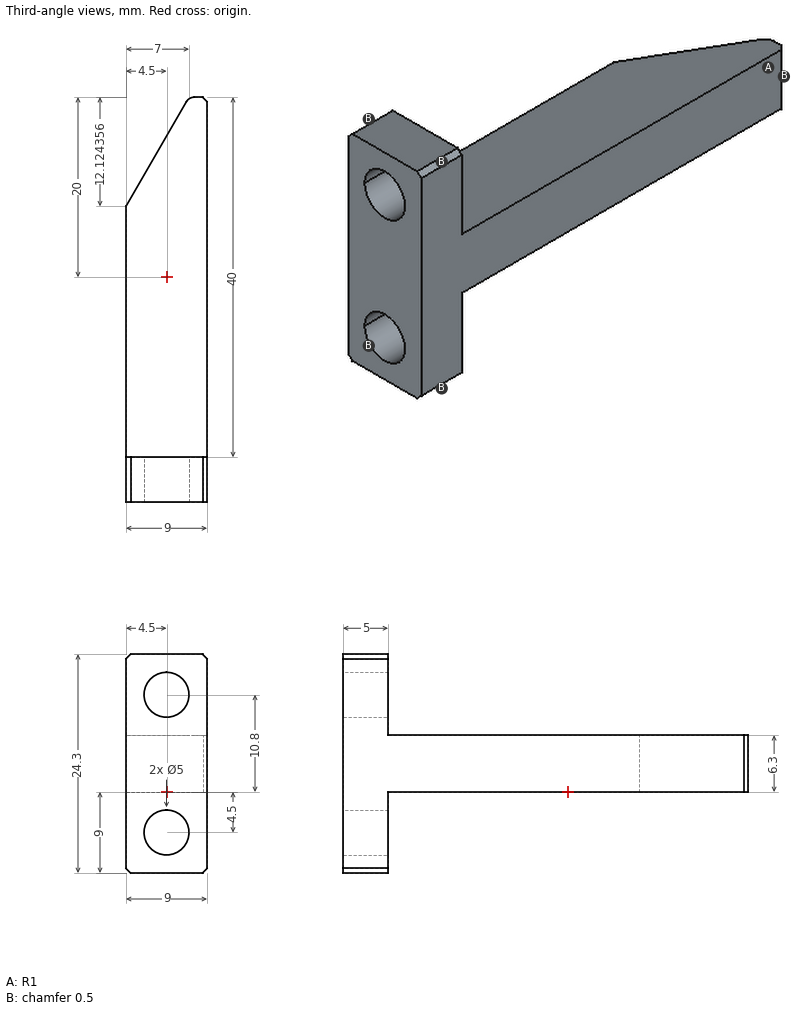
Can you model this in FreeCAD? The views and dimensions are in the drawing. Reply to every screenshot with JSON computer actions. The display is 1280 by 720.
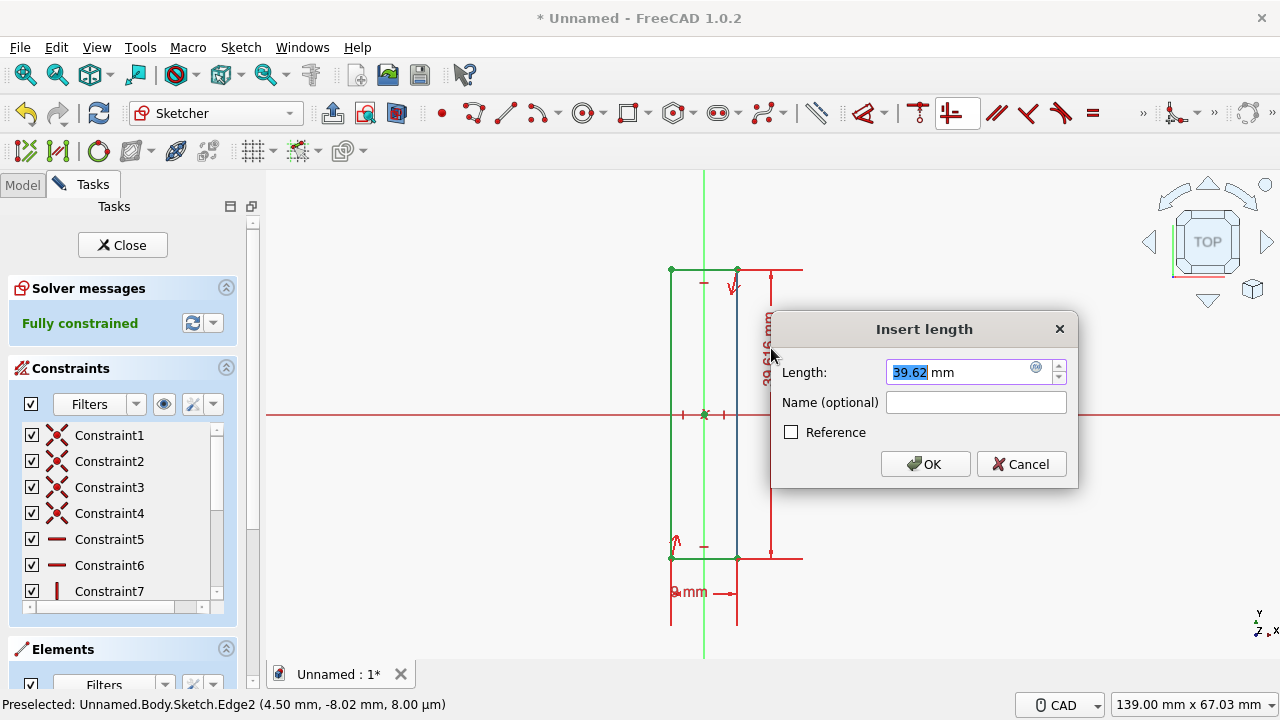
{"action": "type", "text": "40"}
{"action": "key", "text": "Return"}
{"action": "key", "text": "Escape"}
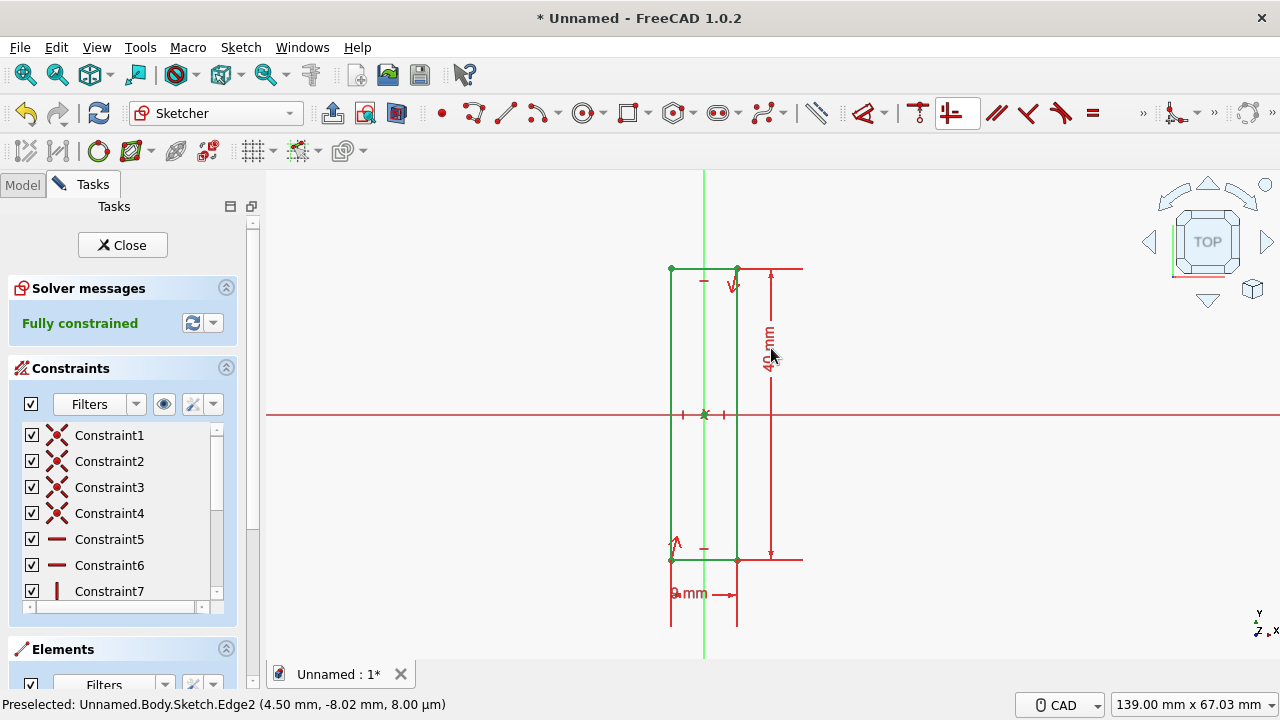
{"action": "left_click", "coordinate": [123, 245]}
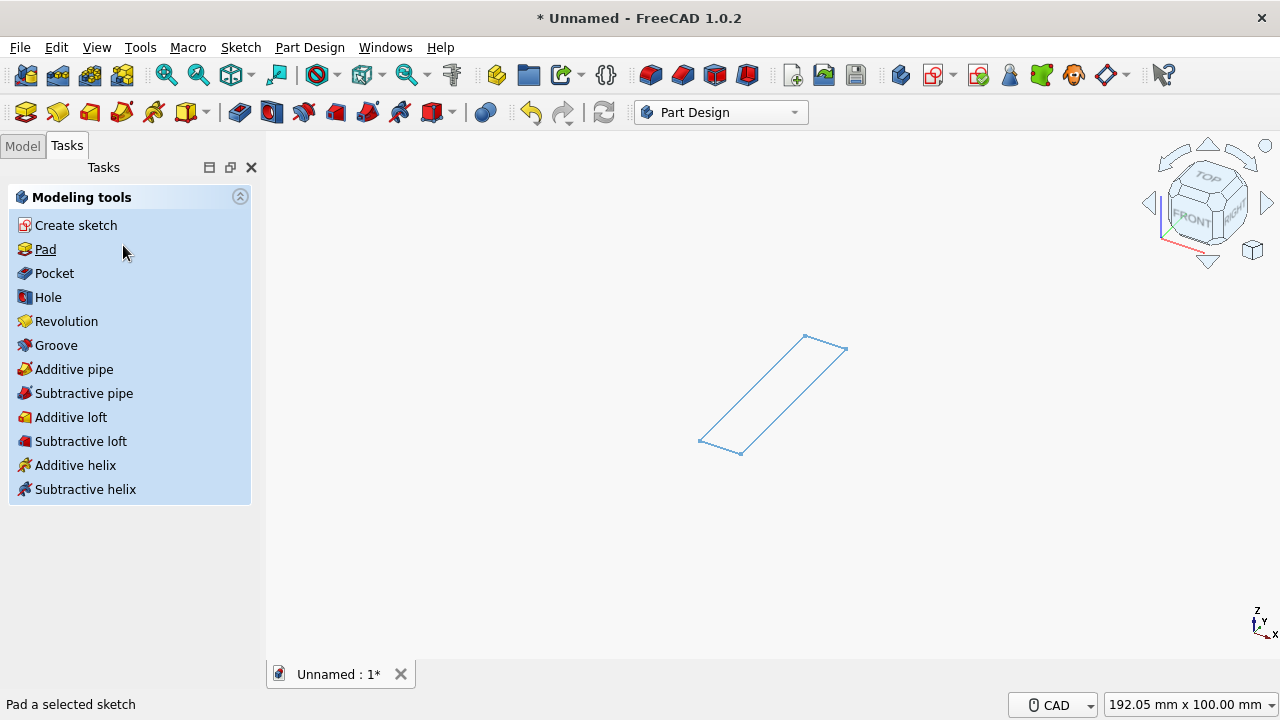
{"action": "left_click", "coordinate": [26, 112]}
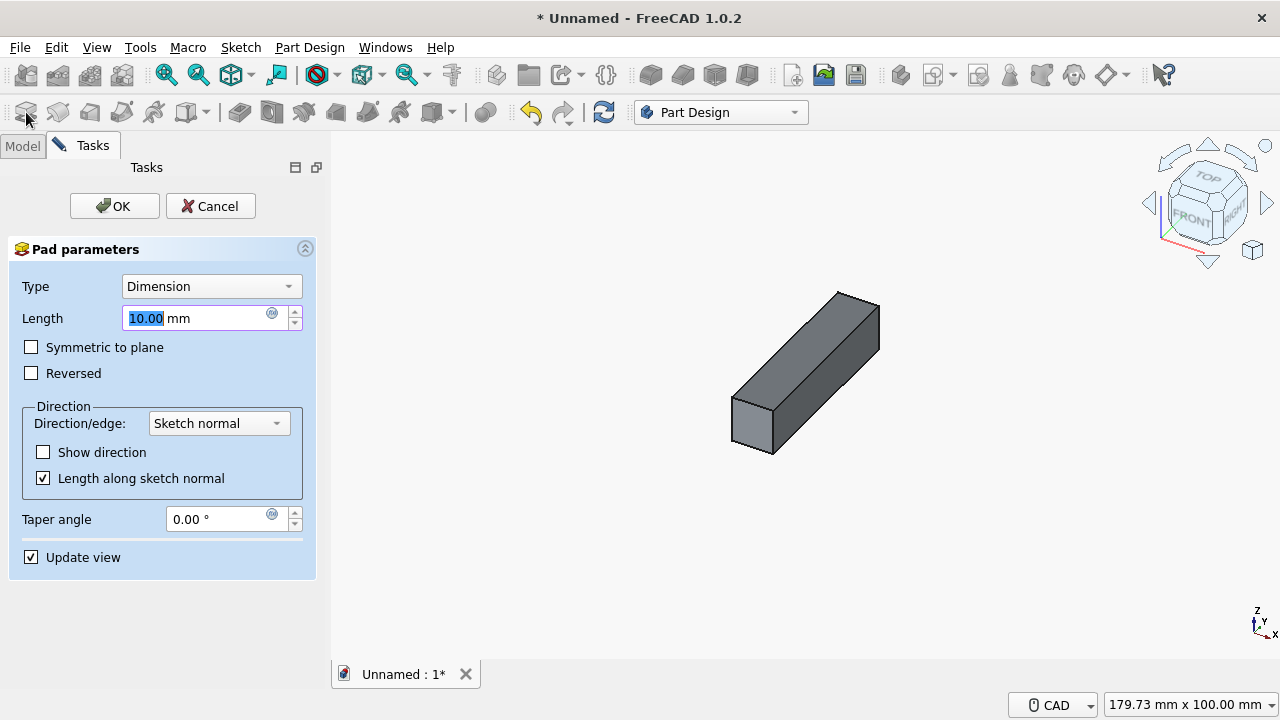
{"action": "type", "text": "6.3"}
{"action": "key", "text": "Tab"}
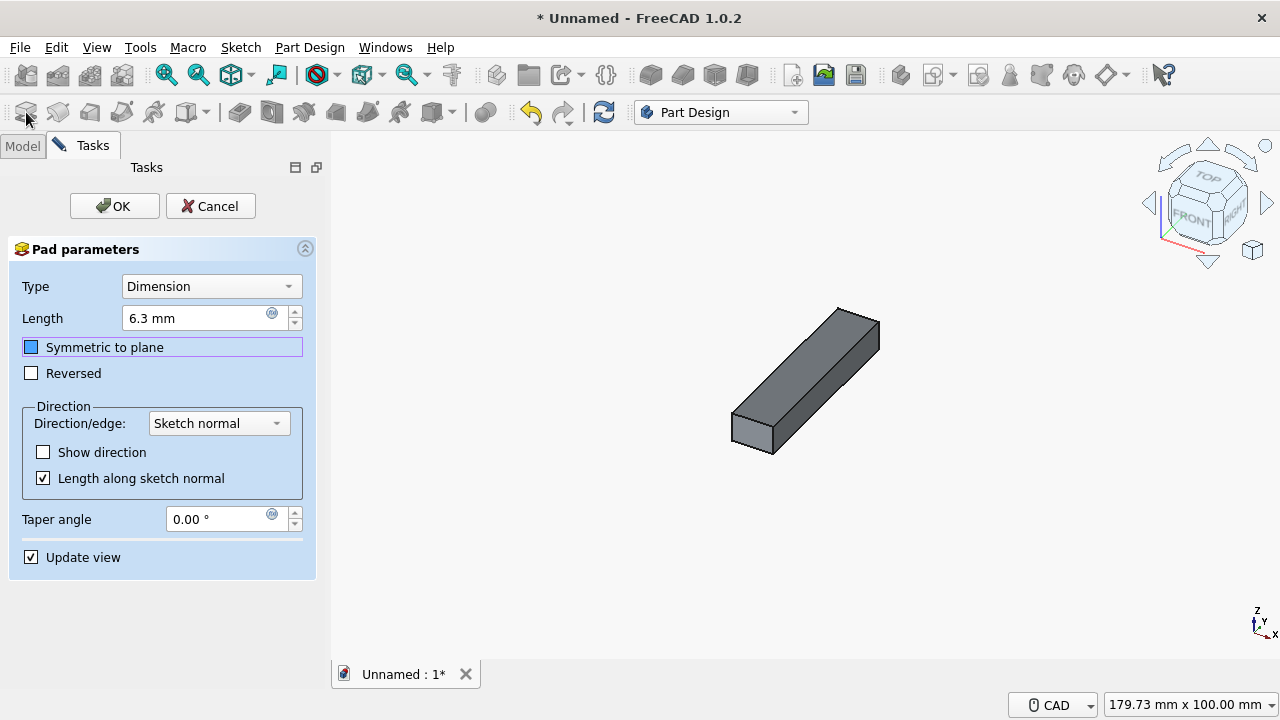
{"action": "left_click", "coordinate": [115, 206]}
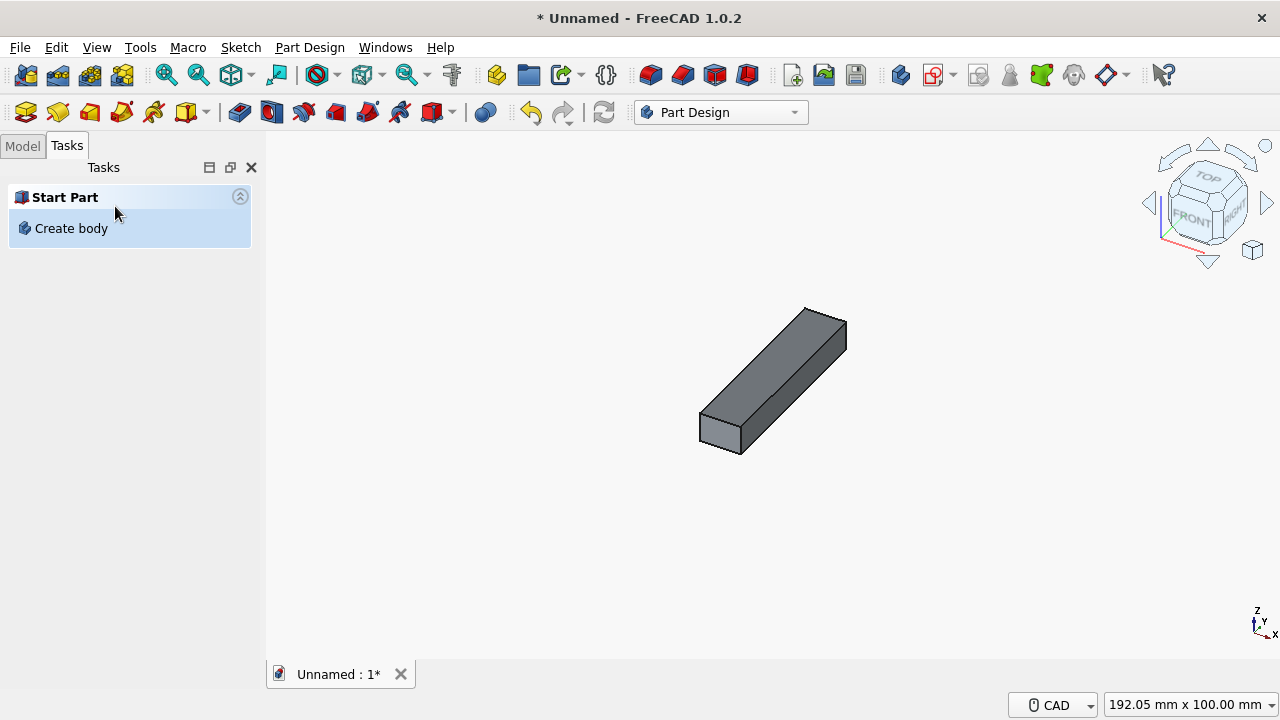
{"action": "left_click", "coordinate": [168, 76]}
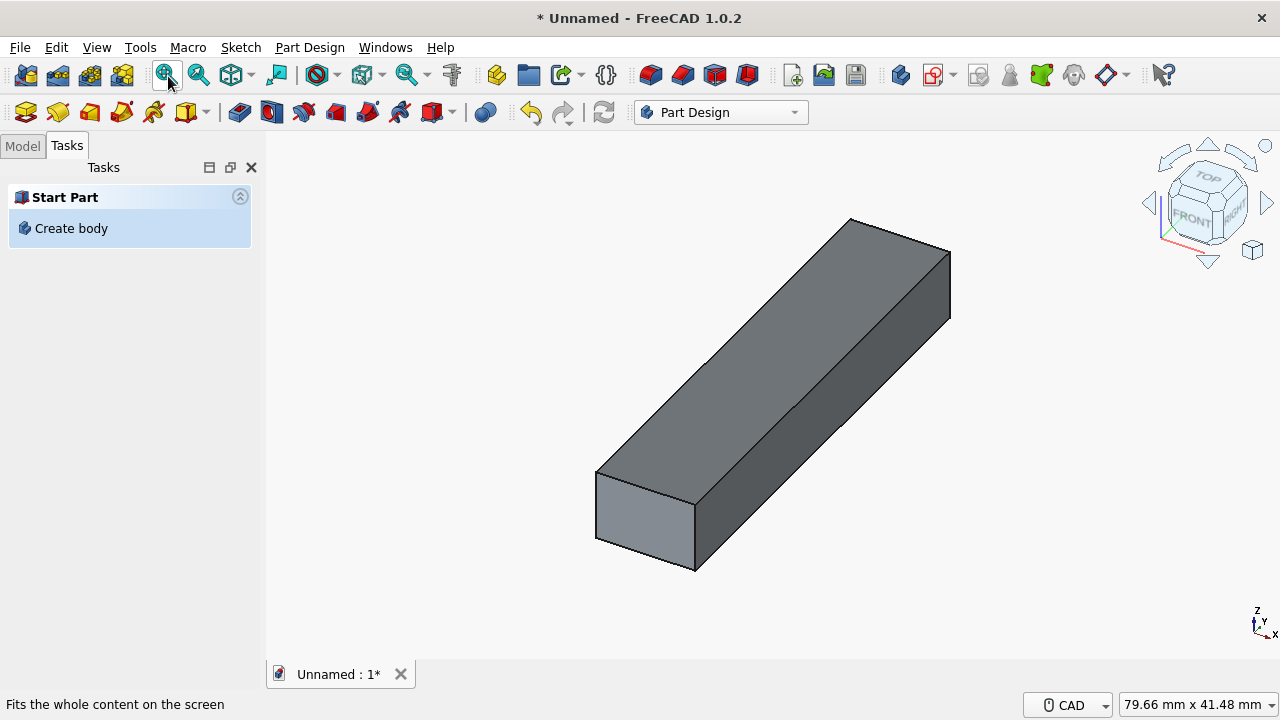
{"action": "left_click", "coordinate": [660, 525]}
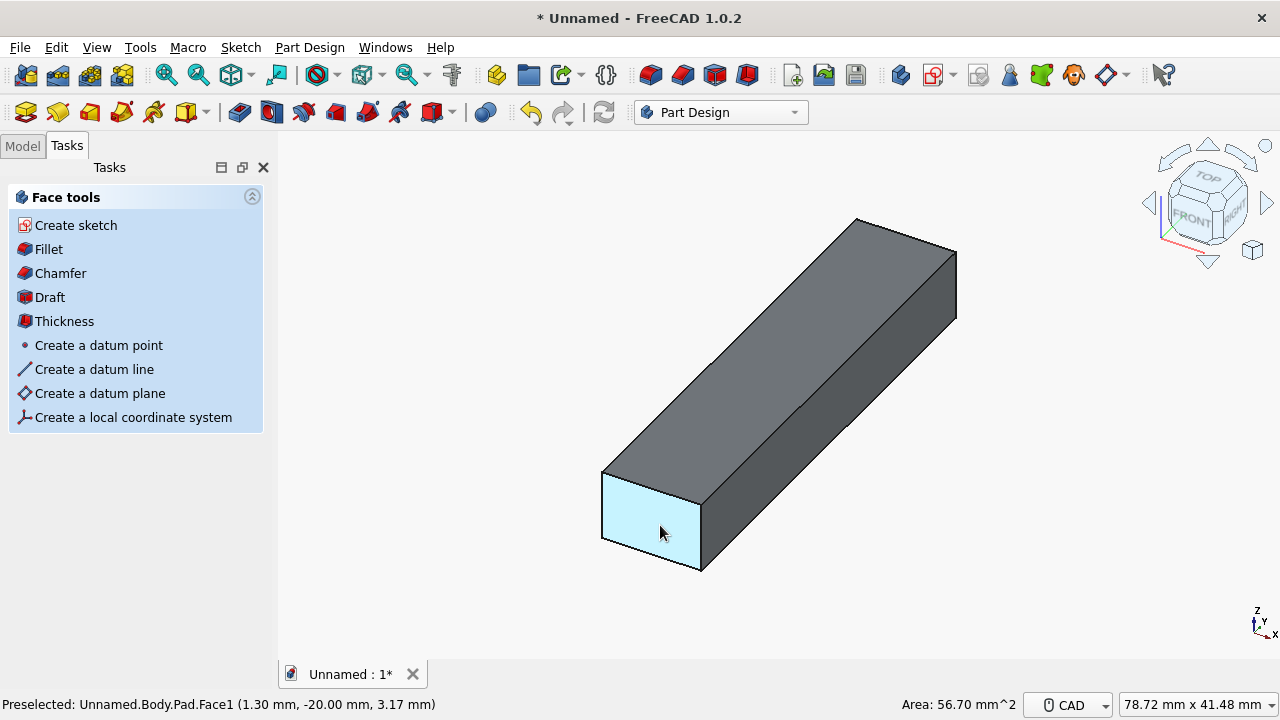
{"action": "left_click", "coordinate": [934, 76]}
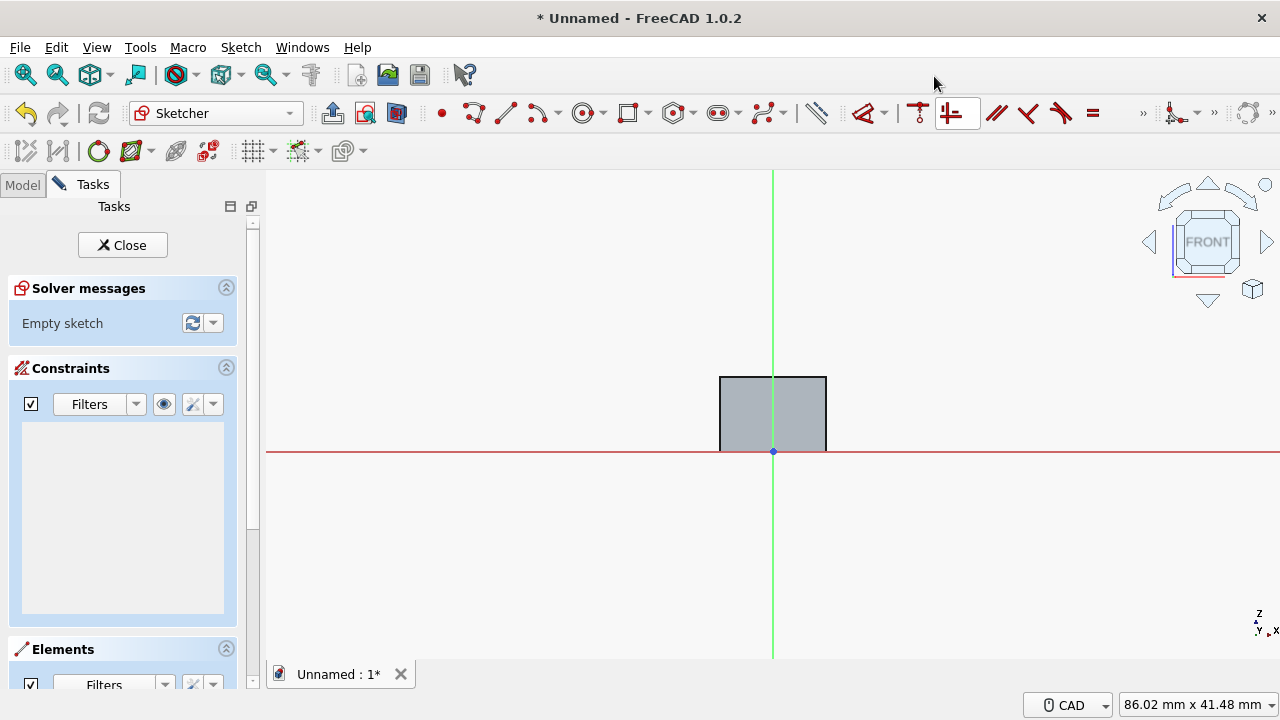
{"action": "left_click", "coordinate": [628, 114]}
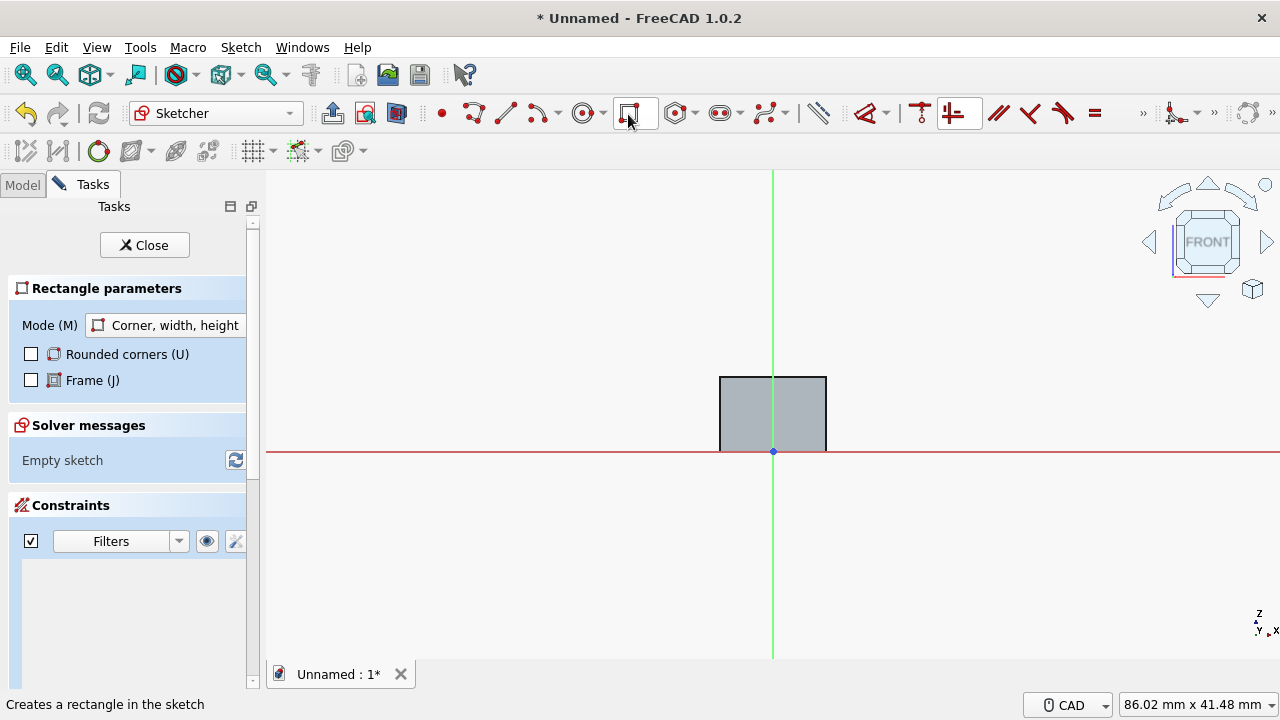
{"action": "left_click", "coordinate": [720, 271]}
{"action": "left_click", "coordinate": [826, 558]}
{"action": "key", "text": "Escape"}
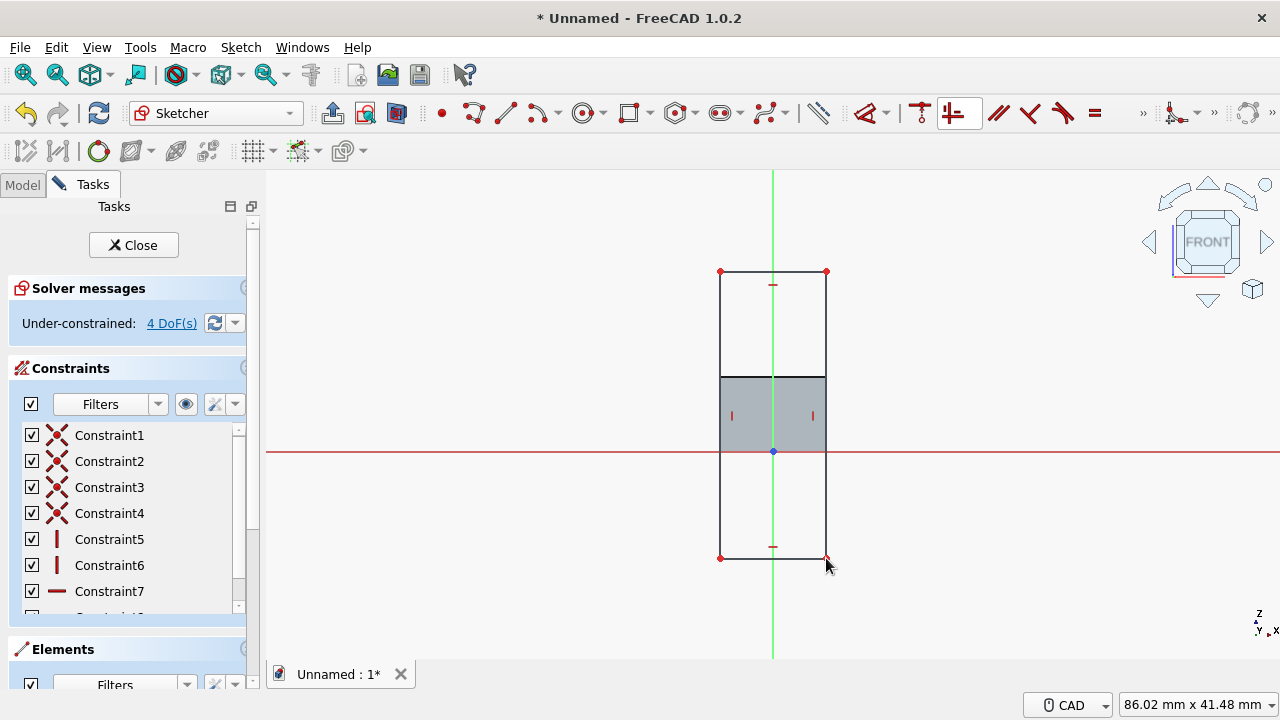
{"action": "left_click", "coordinate": [866, 114]}